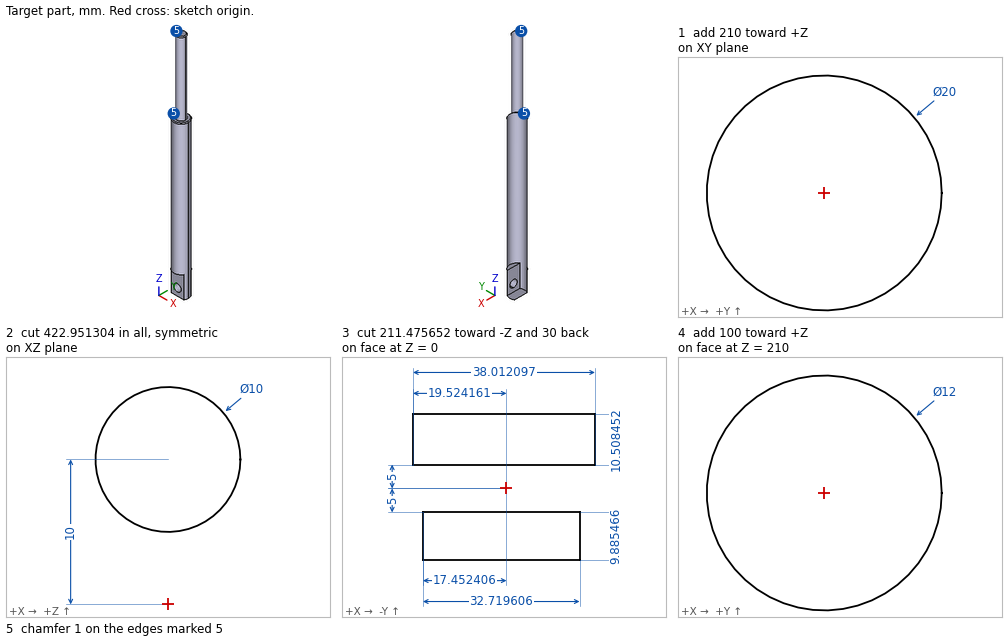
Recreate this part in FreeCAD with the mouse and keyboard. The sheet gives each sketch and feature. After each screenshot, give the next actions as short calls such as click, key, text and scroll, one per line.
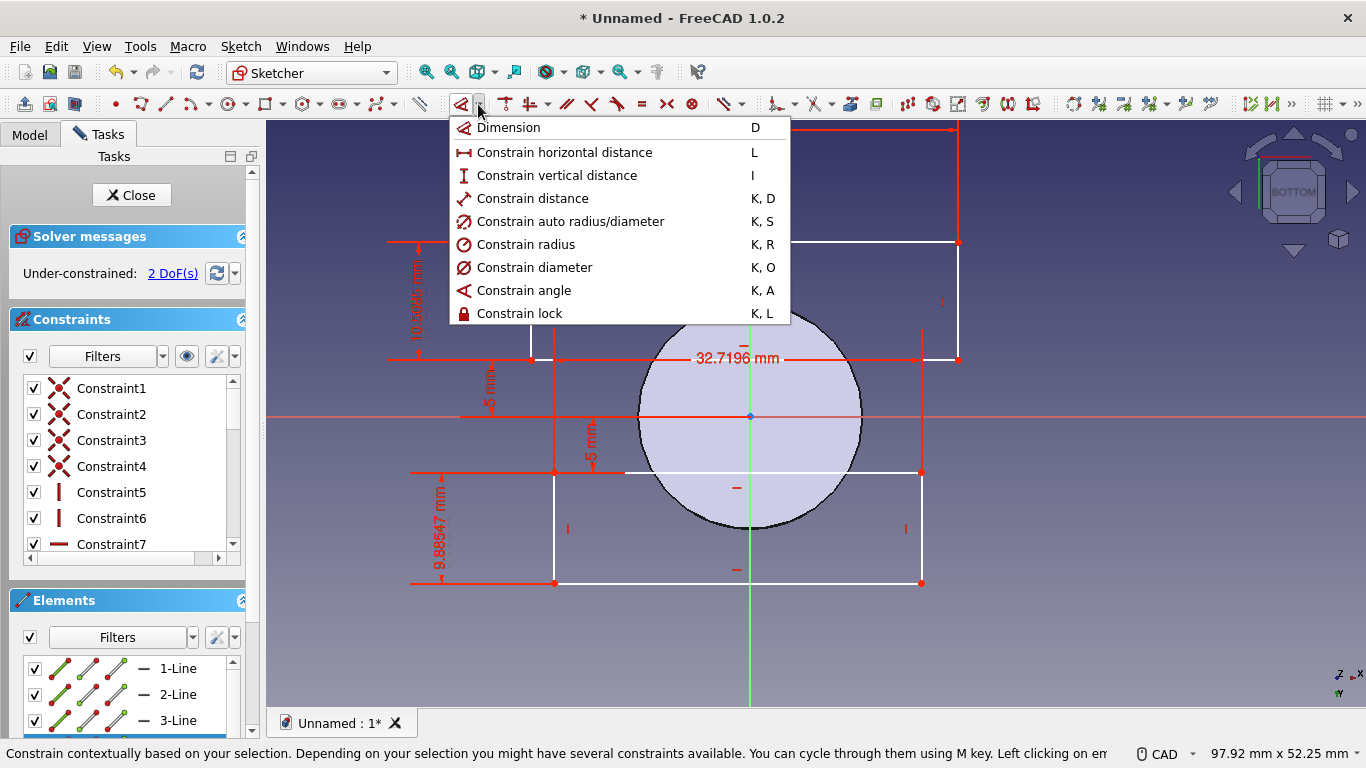
click(620, 152)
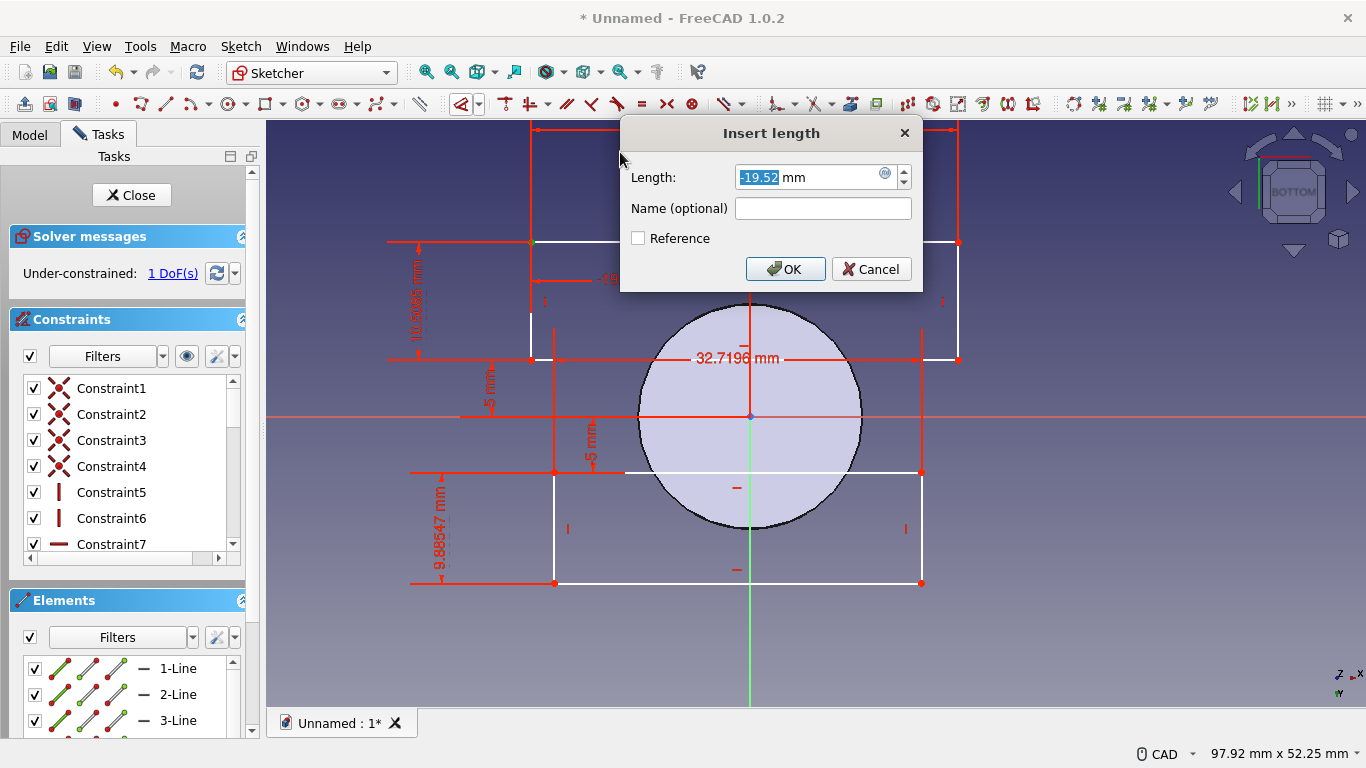
text(-19.524161)
key(Return)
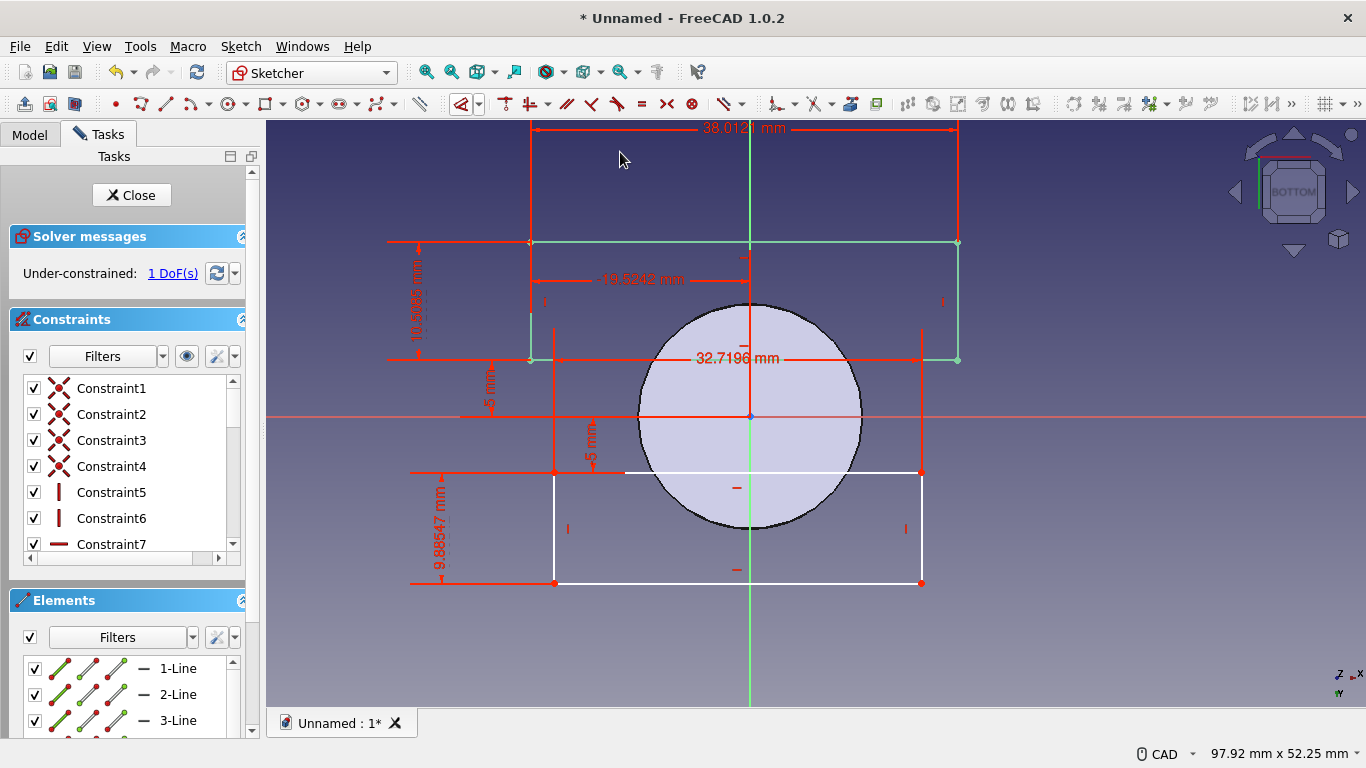
click(554, 473)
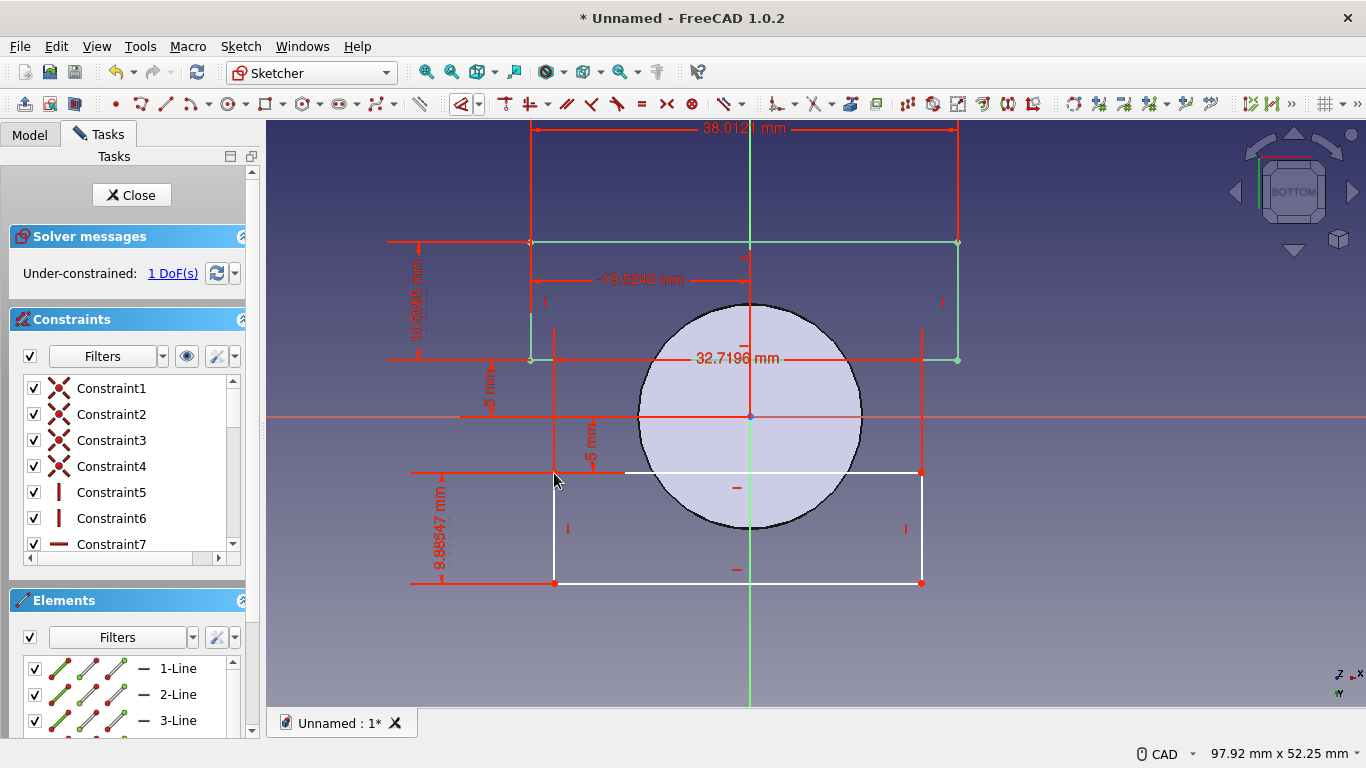
key(l)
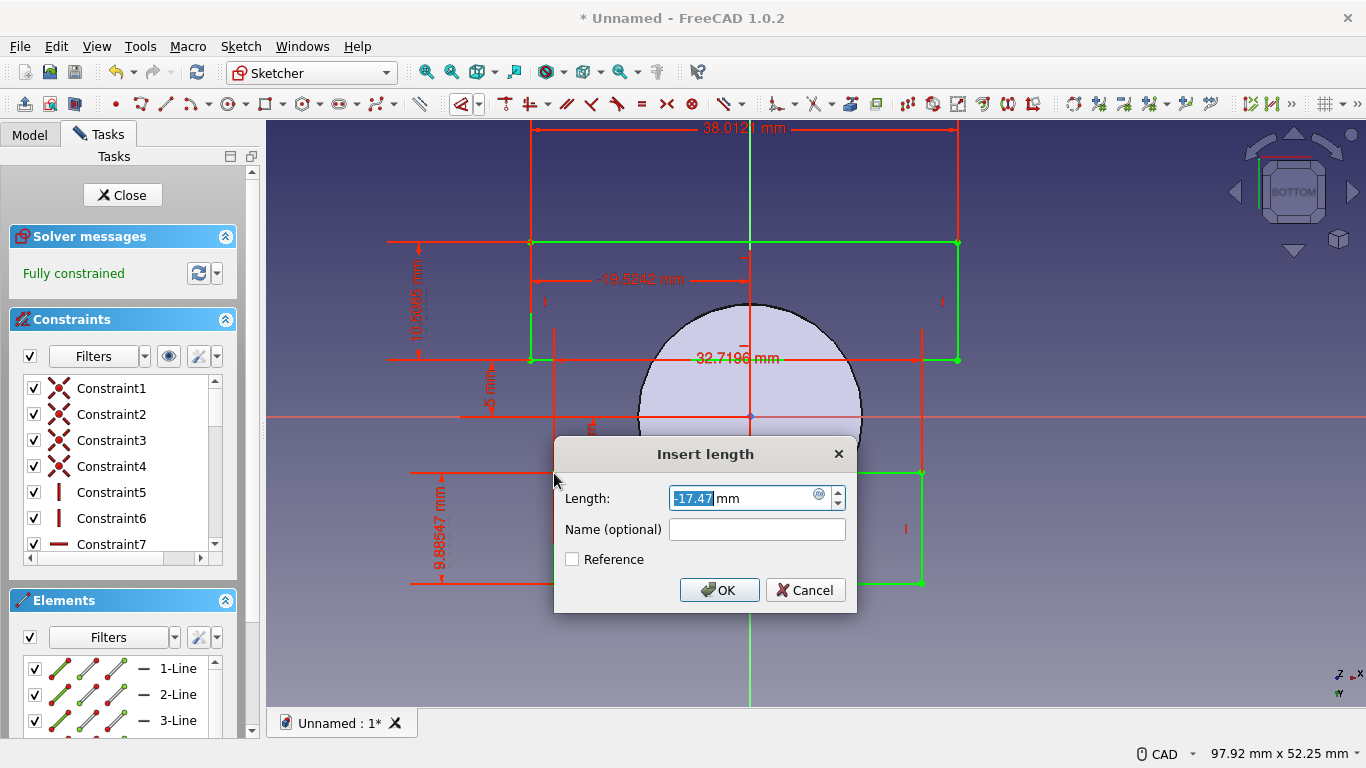
text(-17.452406)
key(Return)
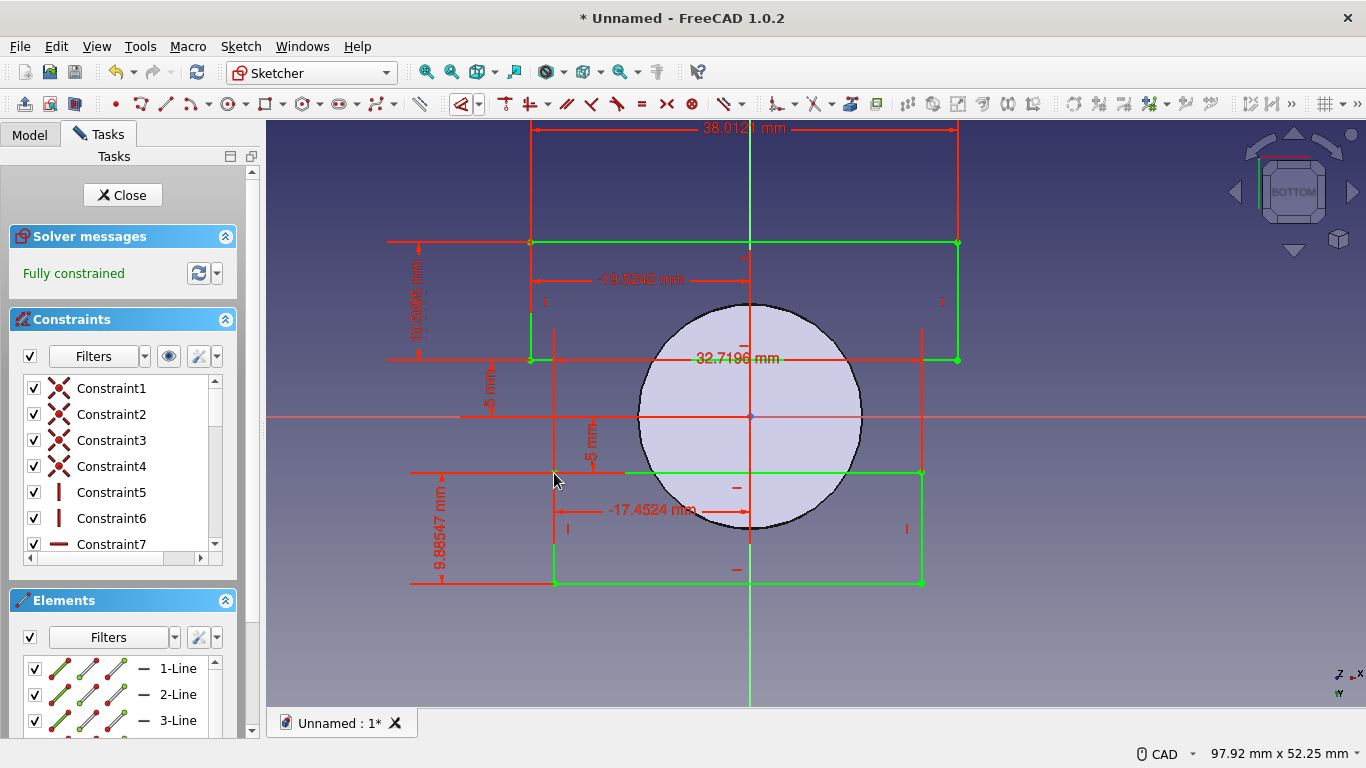
click(123, 195)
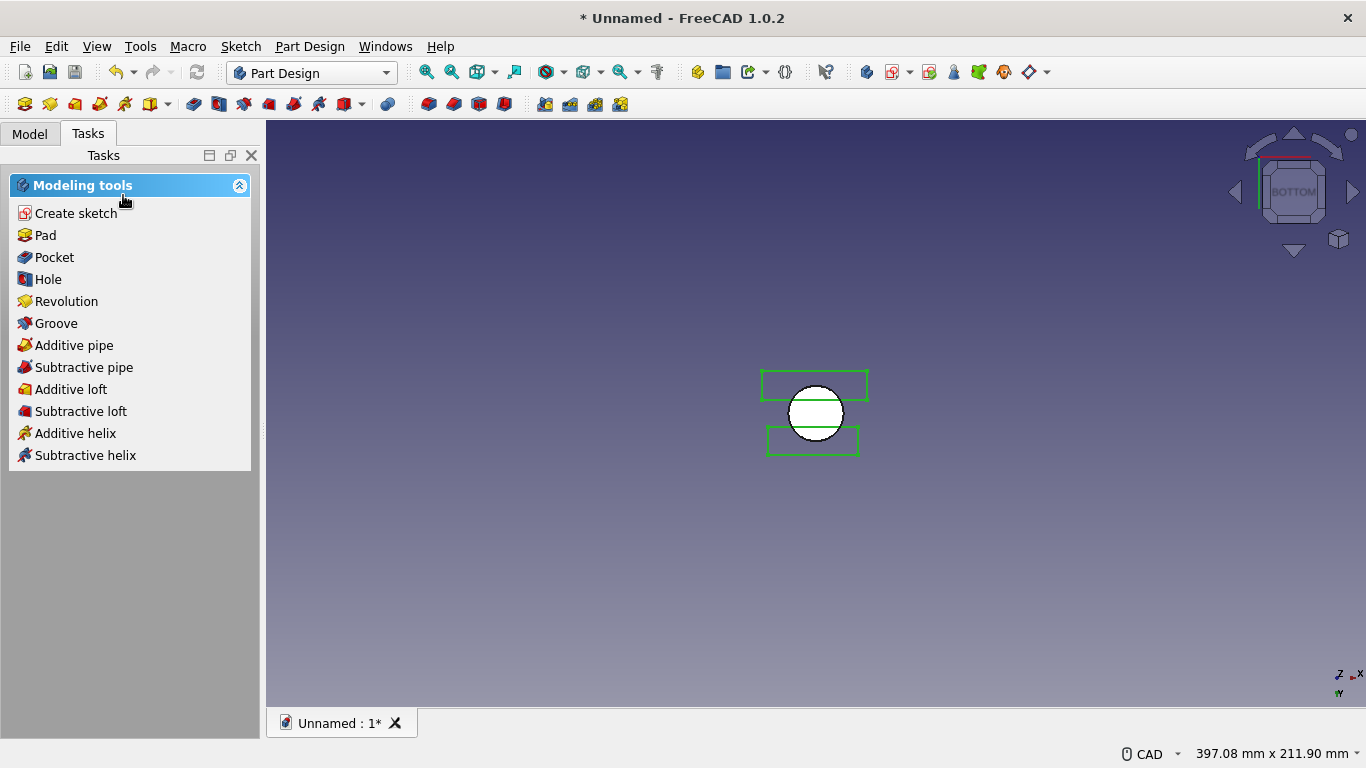
click(194, 104)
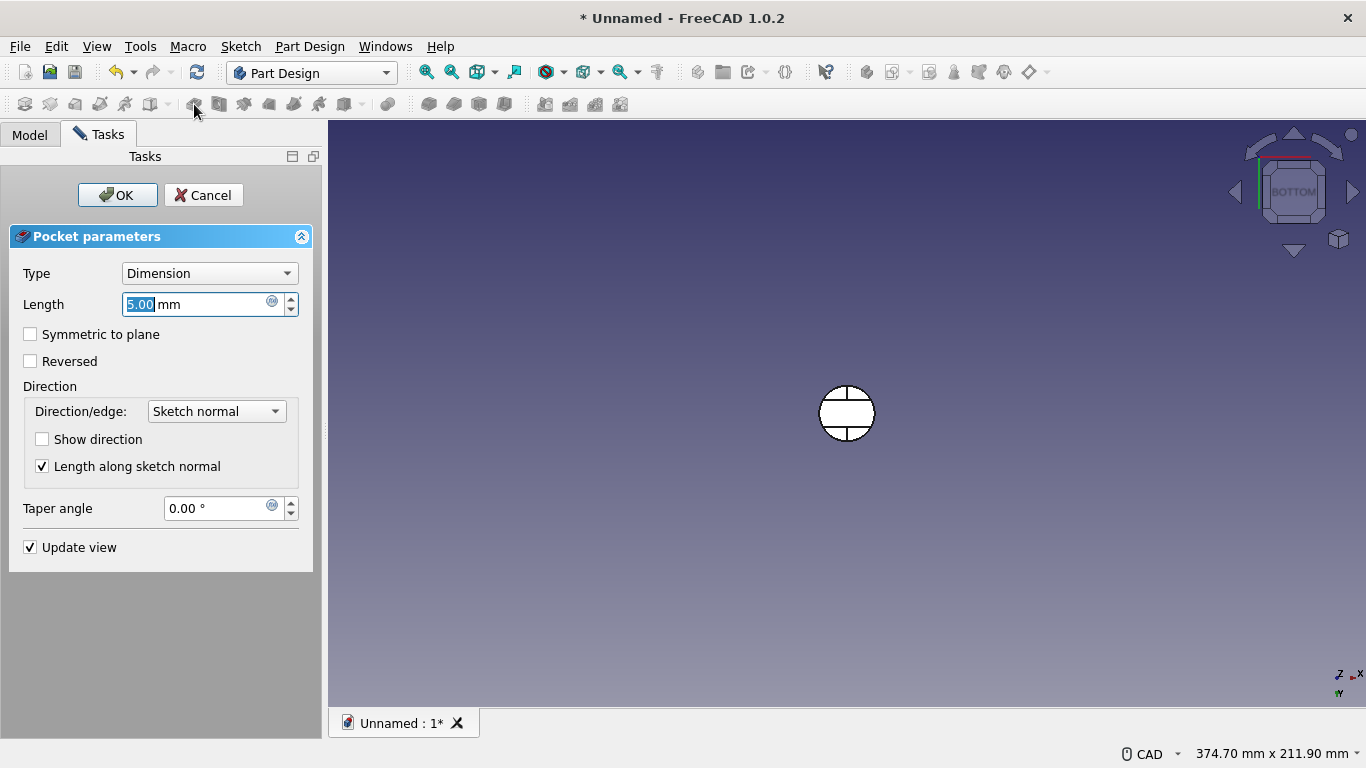
click(210, 274)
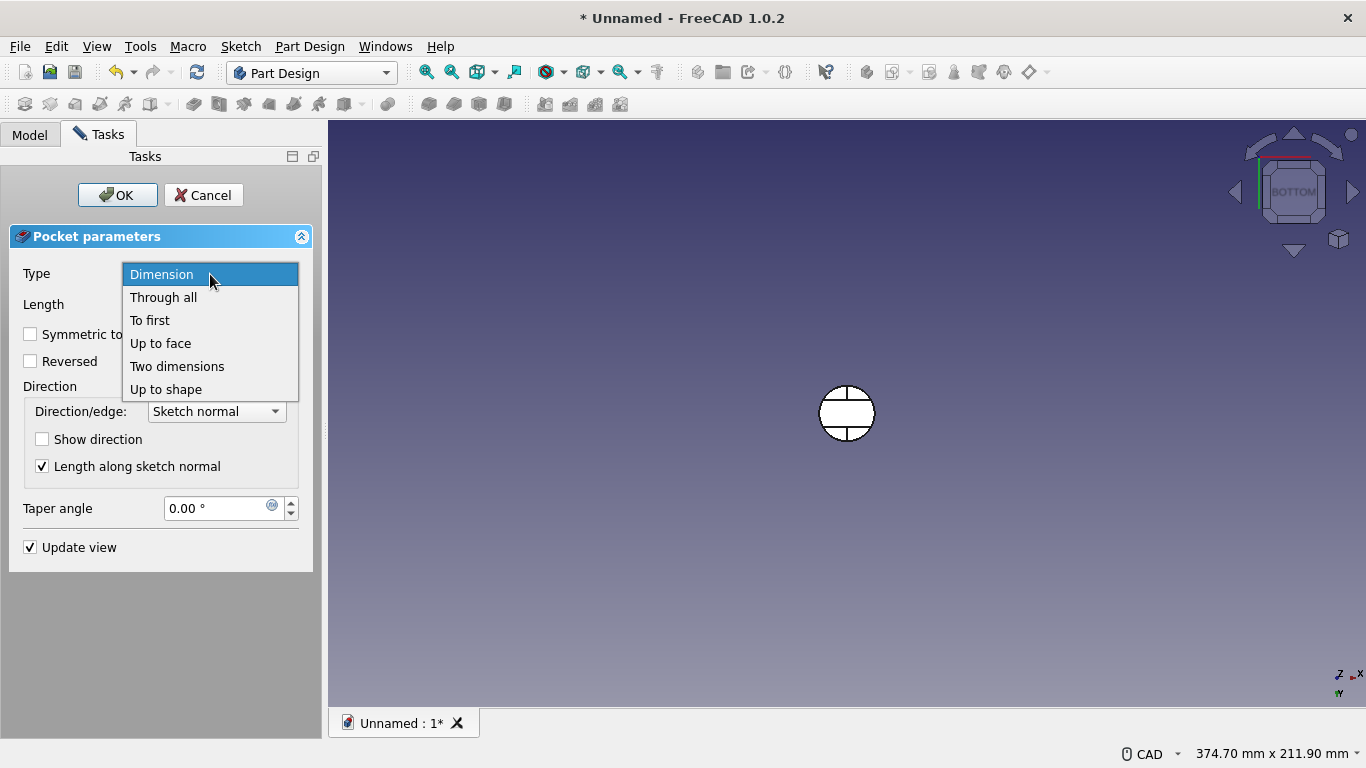
click(208, 366)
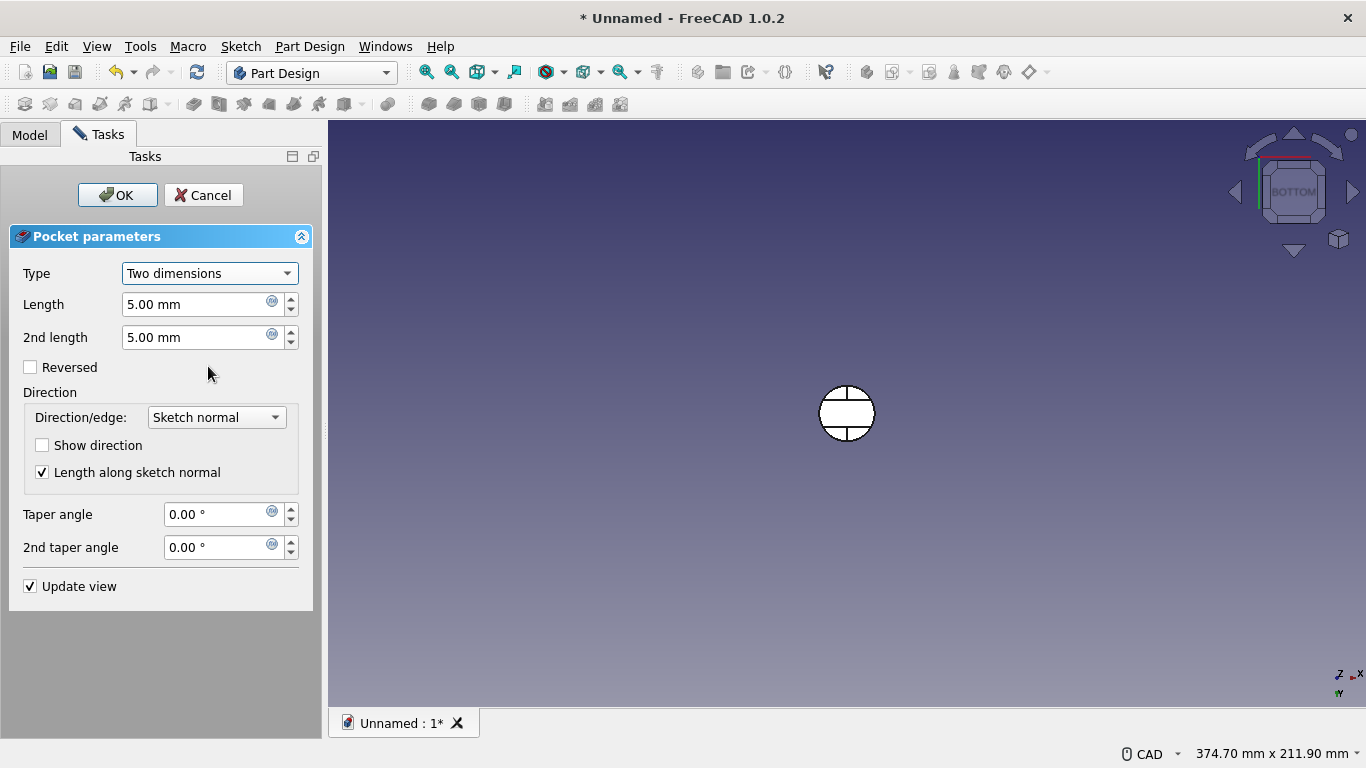
triple_click(204, 304)